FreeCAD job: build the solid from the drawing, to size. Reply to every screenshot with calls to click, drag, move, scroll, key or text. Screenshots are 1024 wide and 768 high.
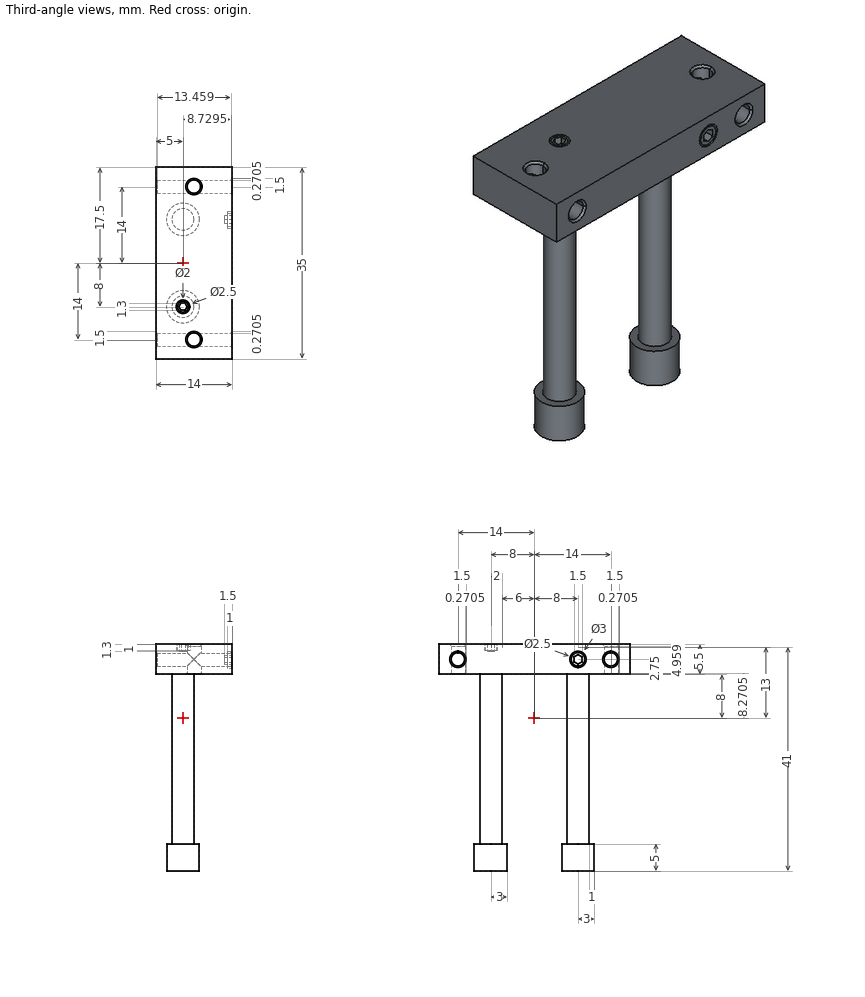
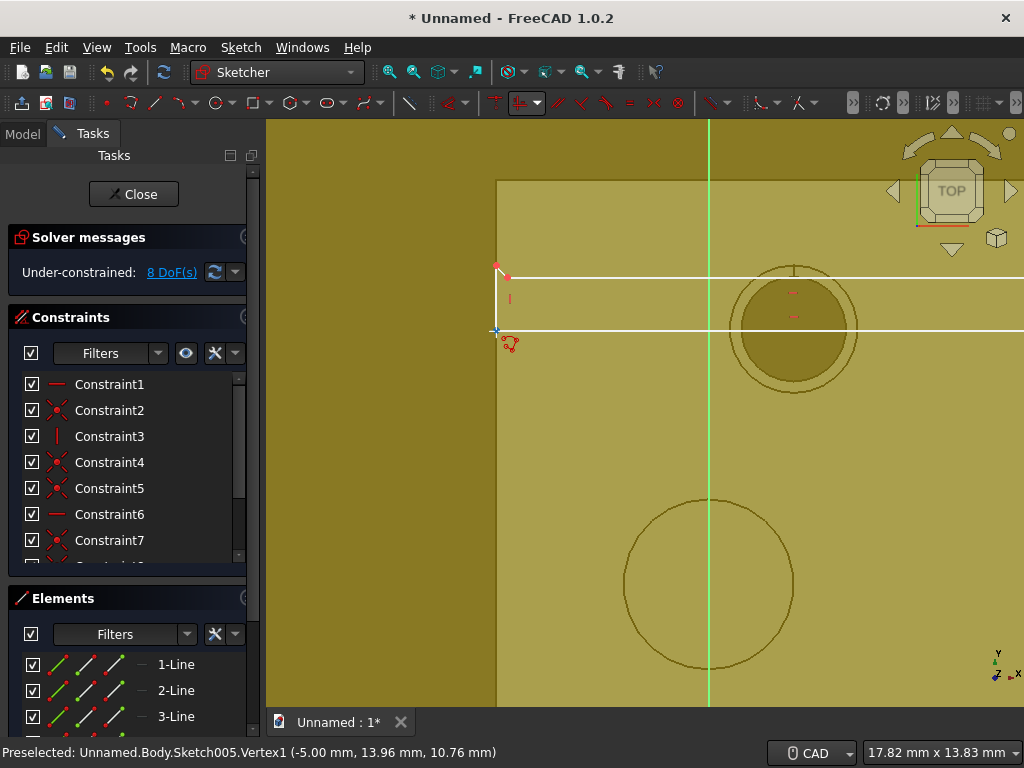
click(156, 104)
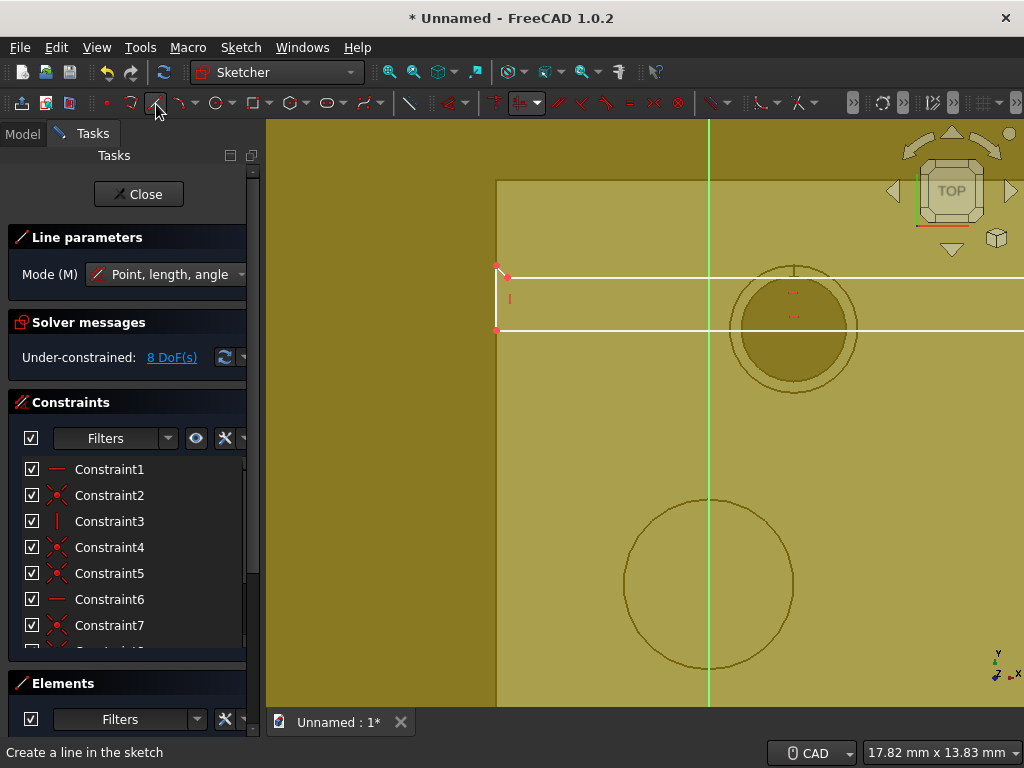
click(436, 329)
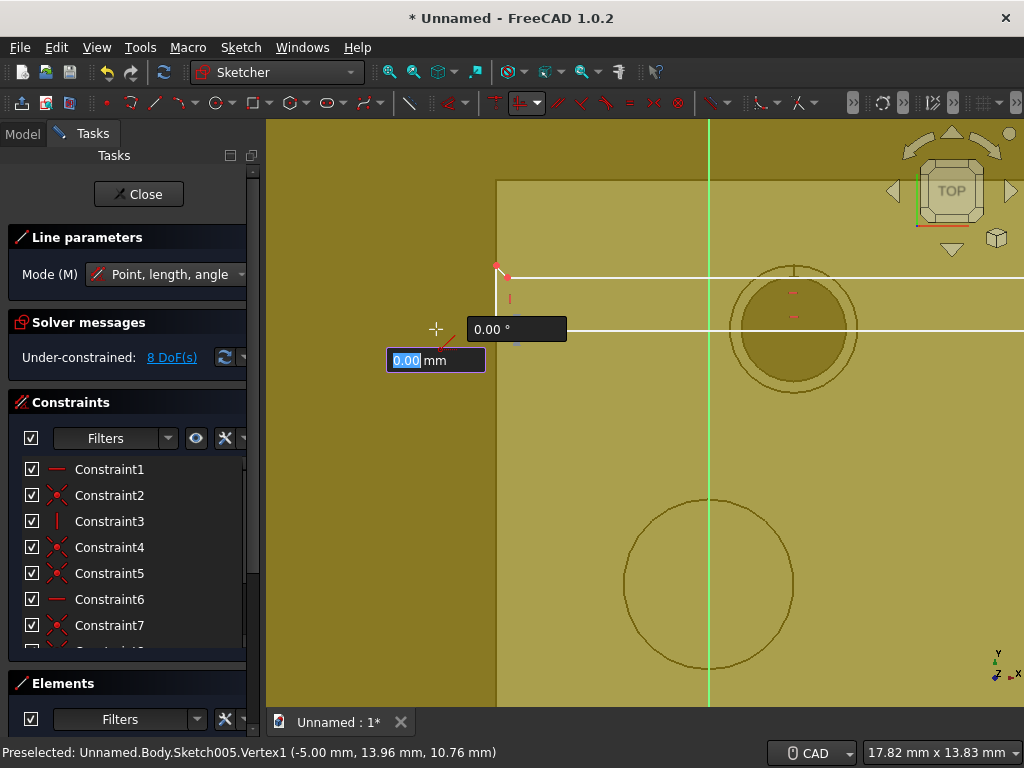
scroll(496, 264, down, 4)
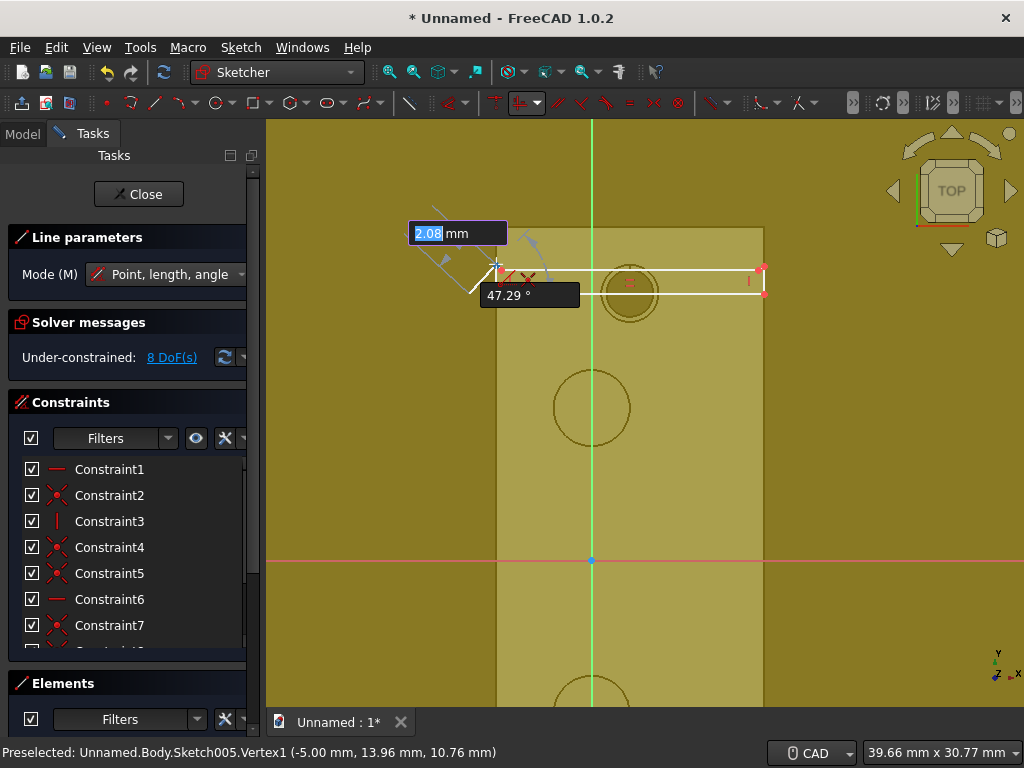
click(389, 293)
key(Escape)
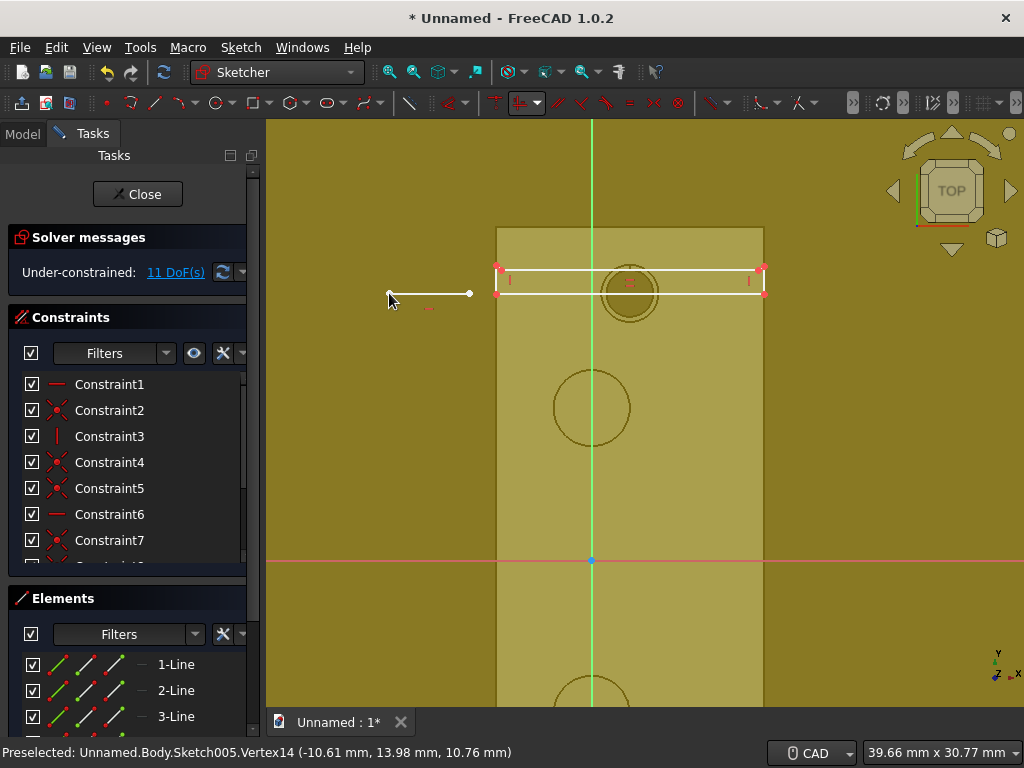
click(445, 294)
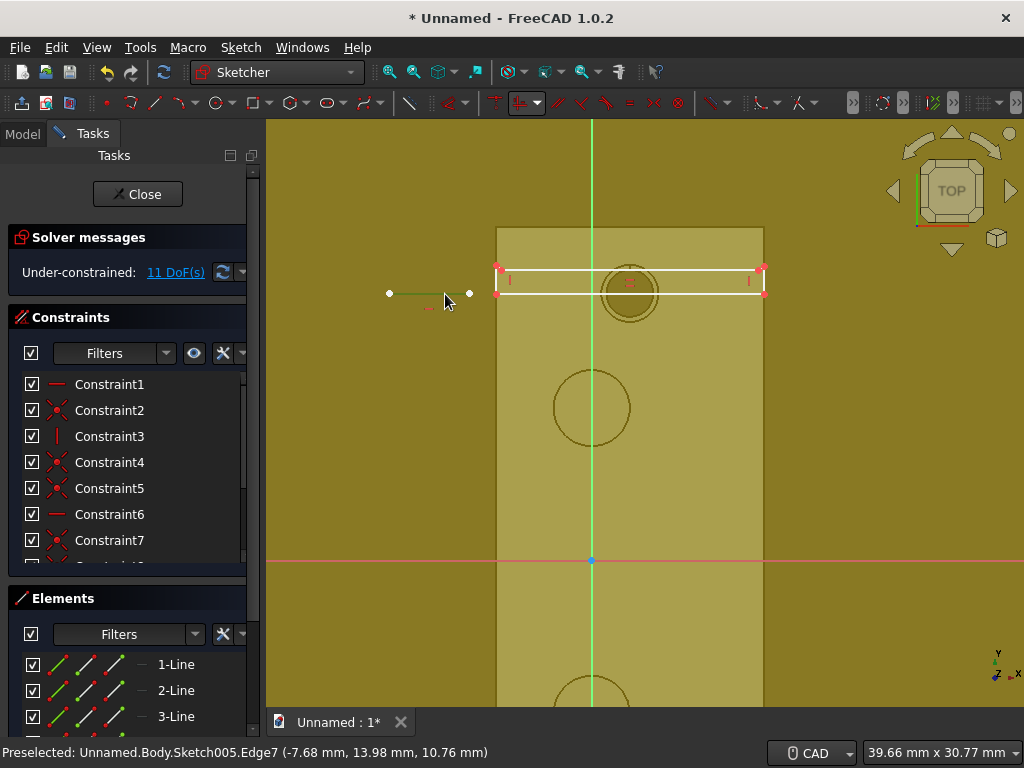
click(410, 104)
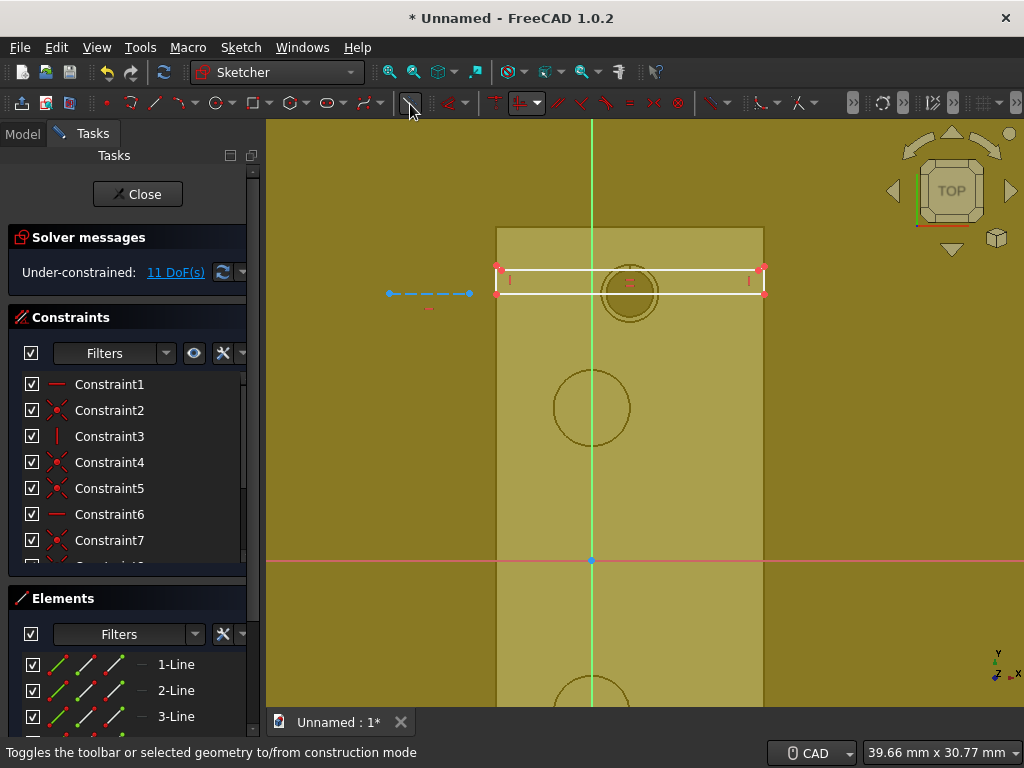
click(448, 104)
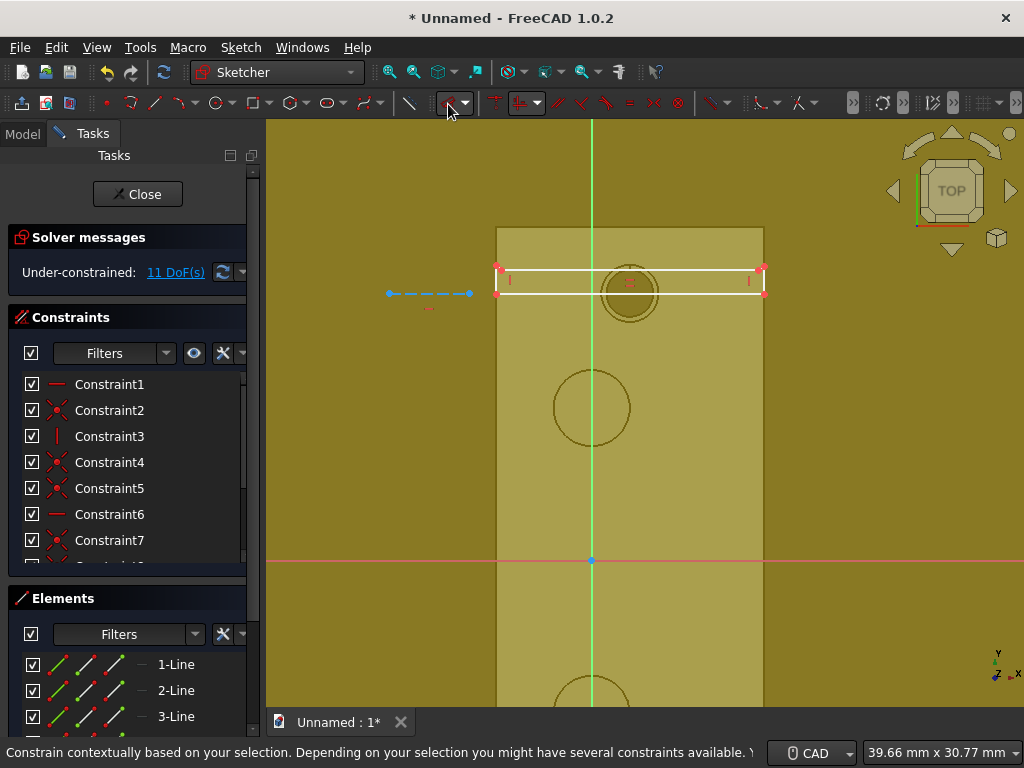
click(577, 294)
click(630, 328)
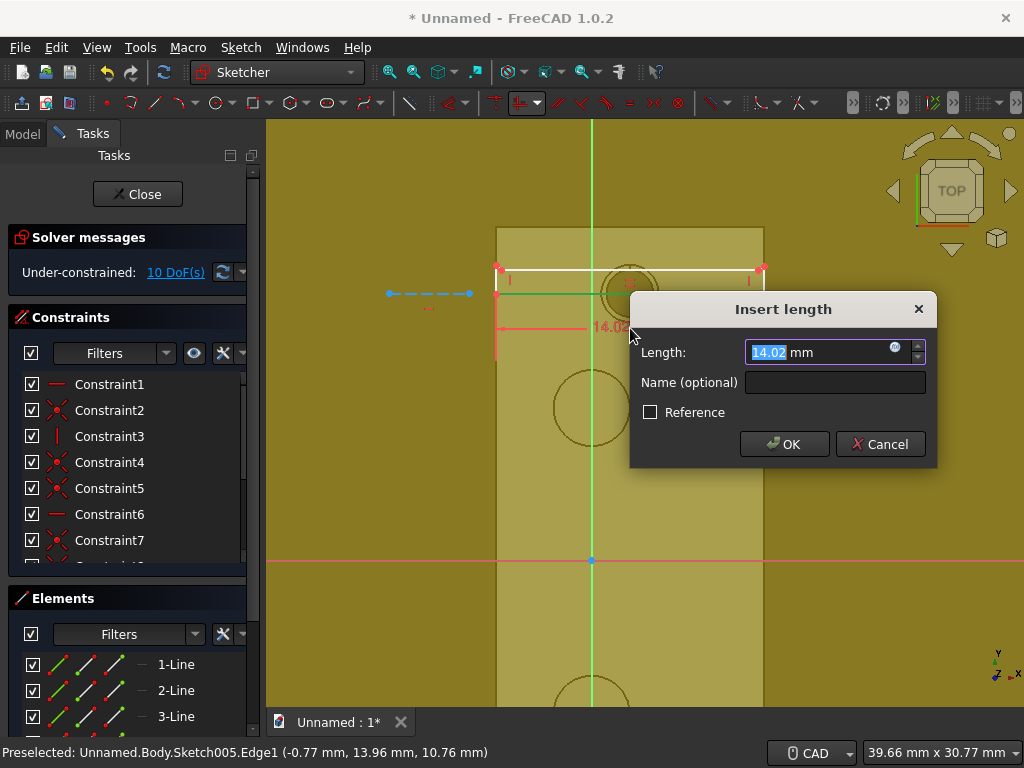
text(14)
key(Return)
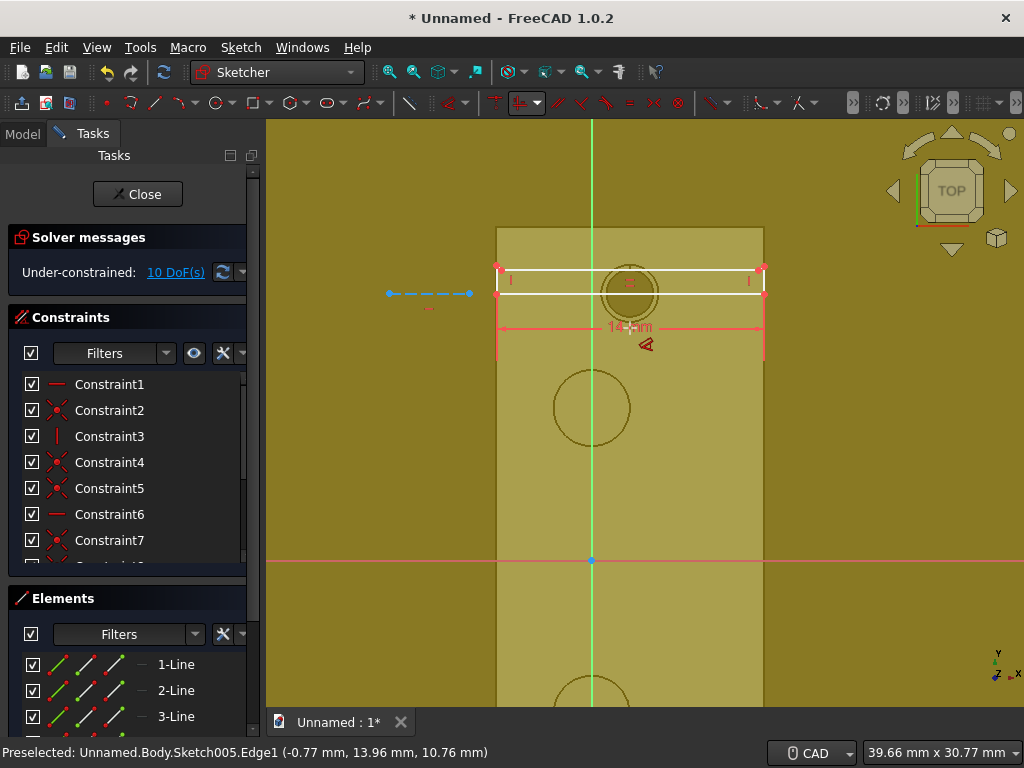
click(497, 294)
click(544, 595)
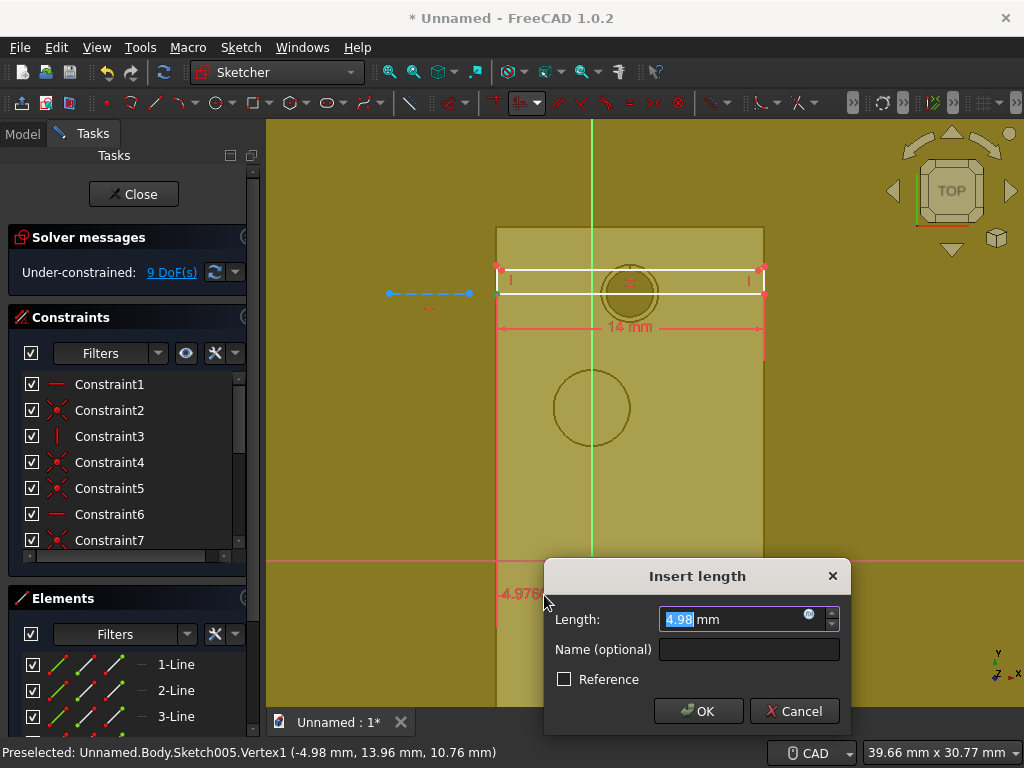
text(5)
key(Return)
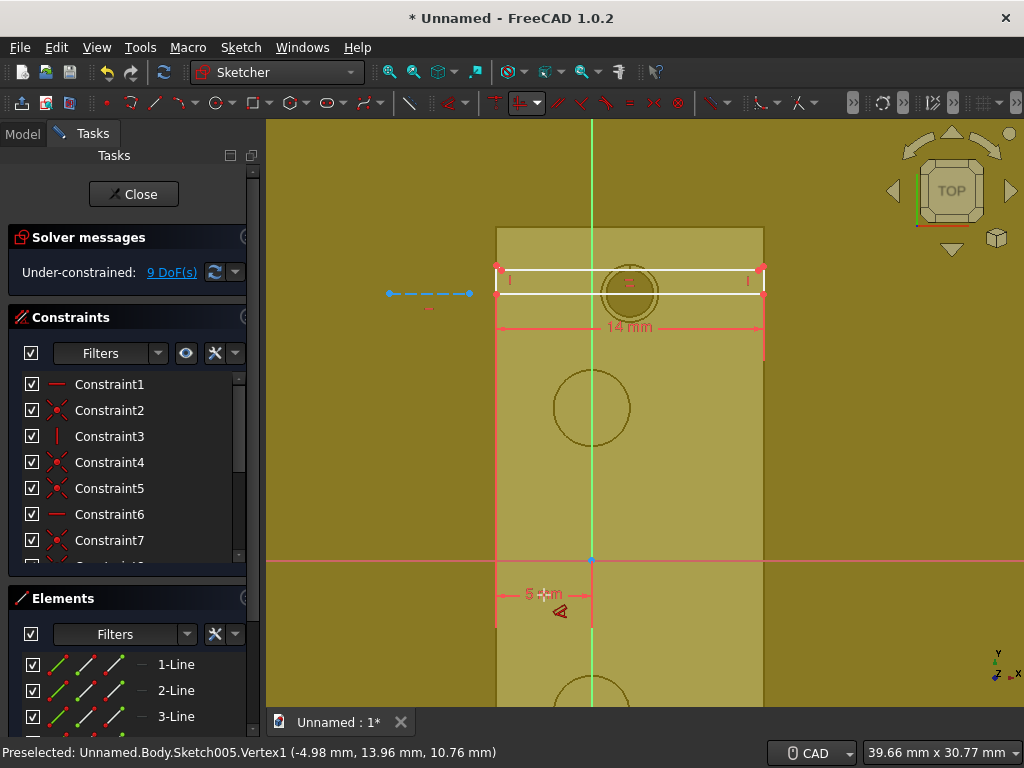
scroll(764, 283, up, 2)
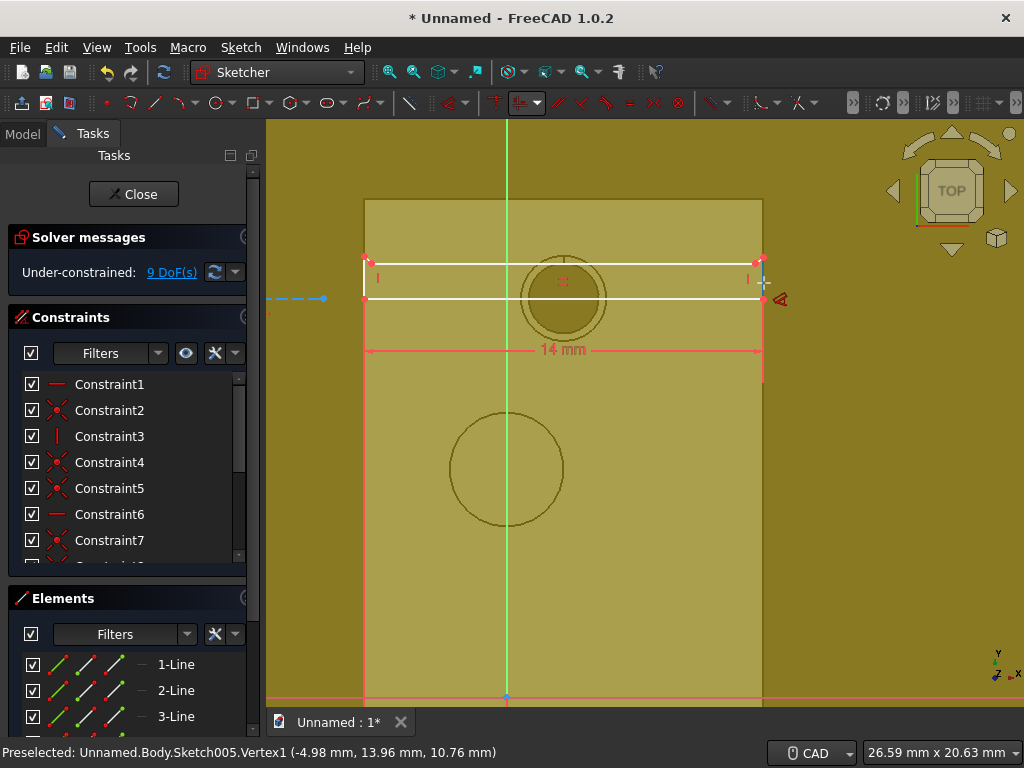
click(763, 283)
click(797, 279)